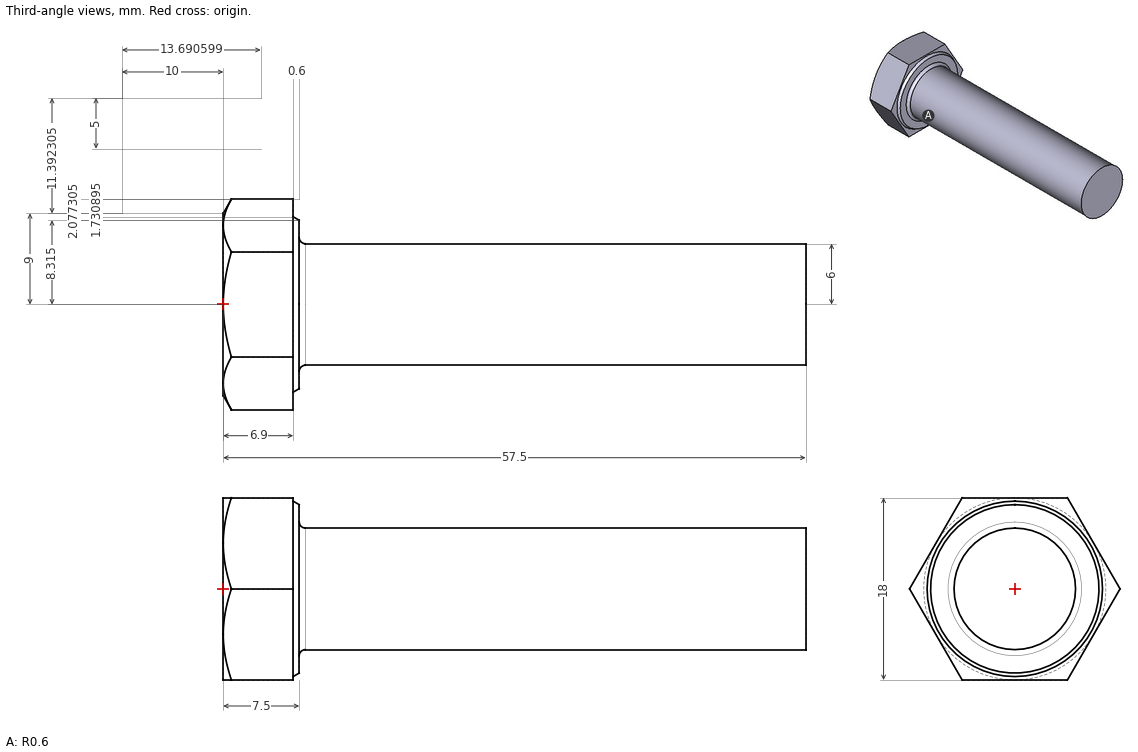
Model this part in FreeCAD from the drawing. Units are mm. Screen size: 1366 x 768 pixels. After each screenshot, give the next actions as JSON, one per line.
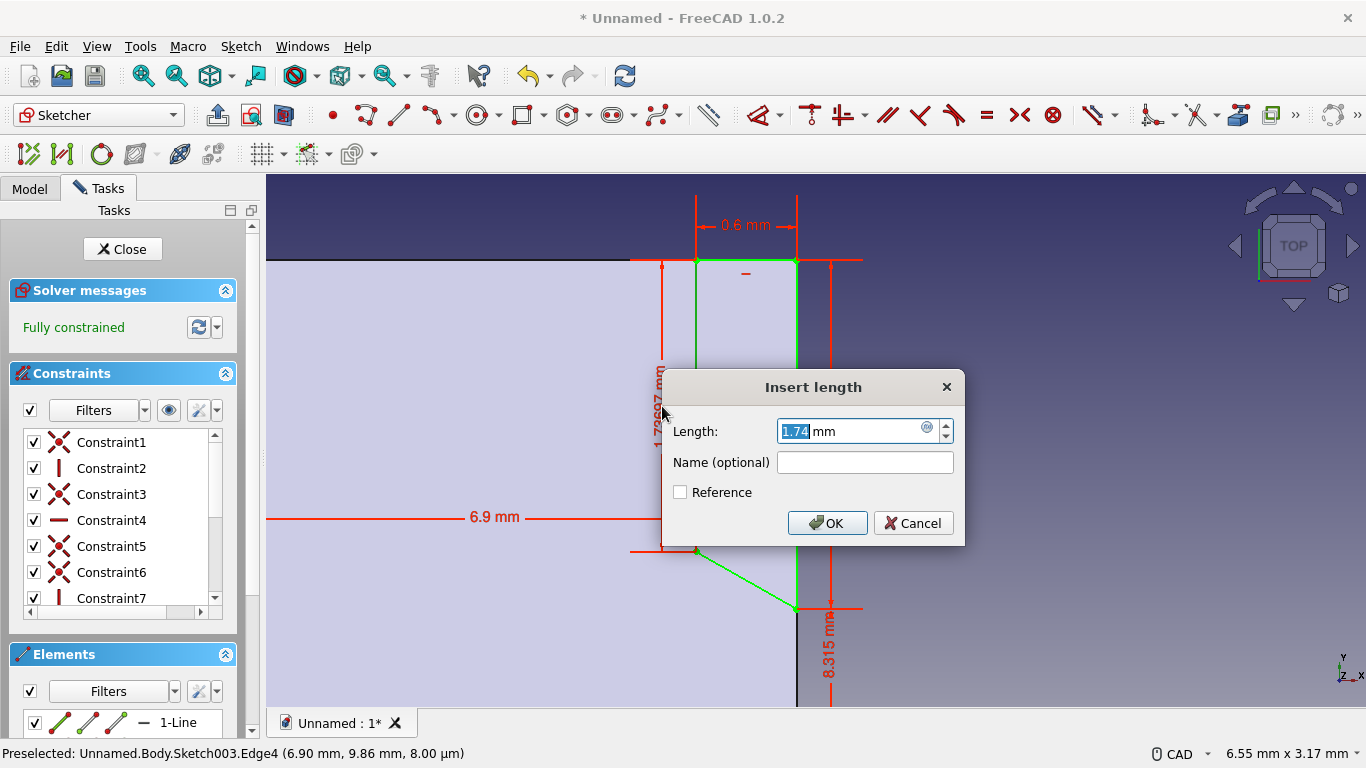
{"action": "type", "text": "1.730895"}
{"action": "key", "text": "Return"}
{"action": "key", "text": "Escape"}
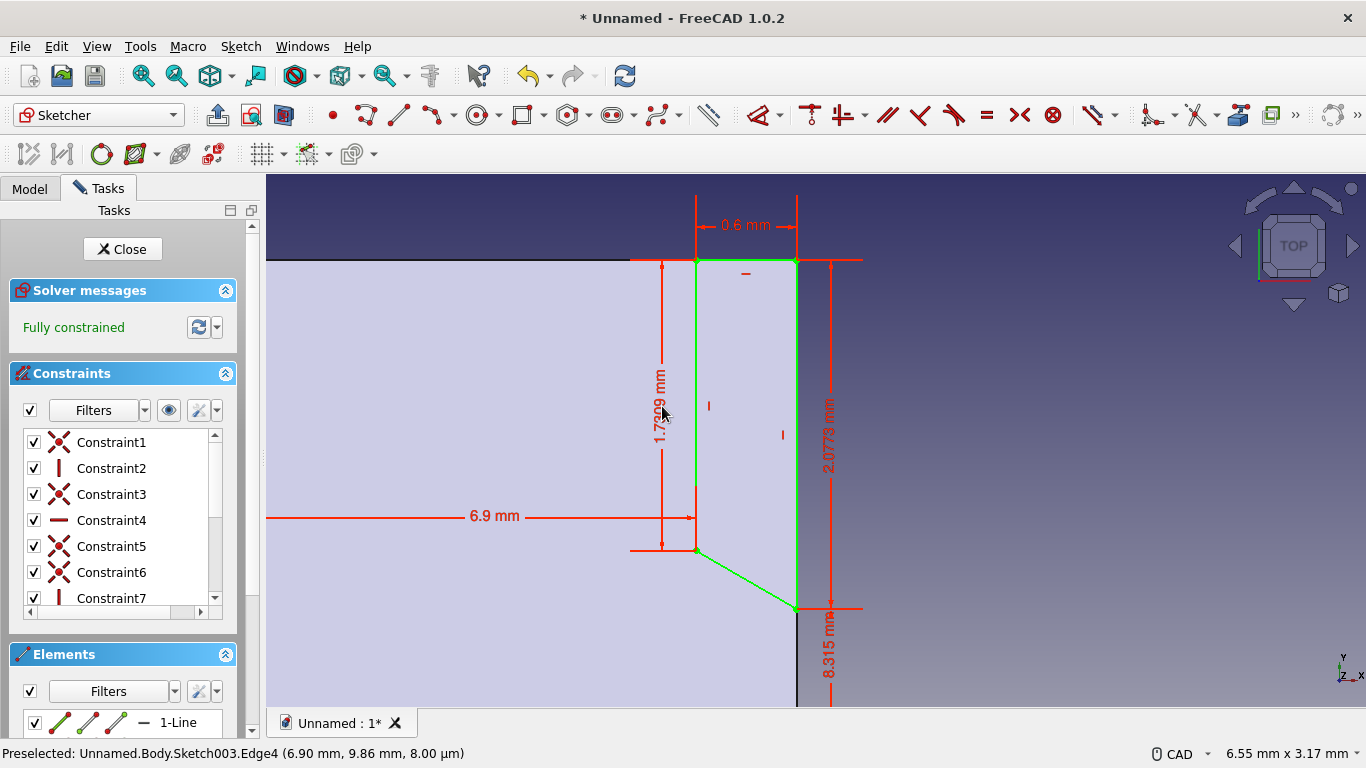
{"action": "left_click", "coordinate": [123, 249]}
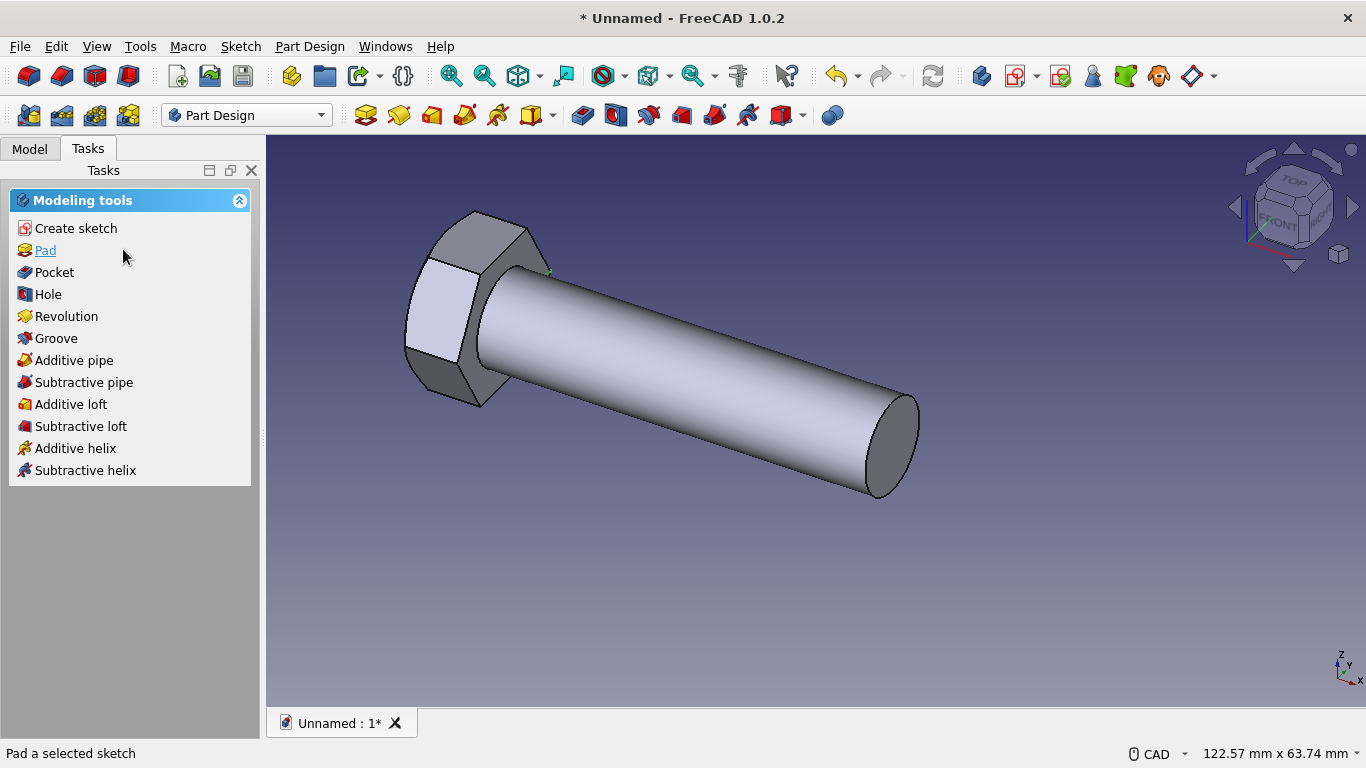
{"action": "left_click", "coordinate": [649, 116]}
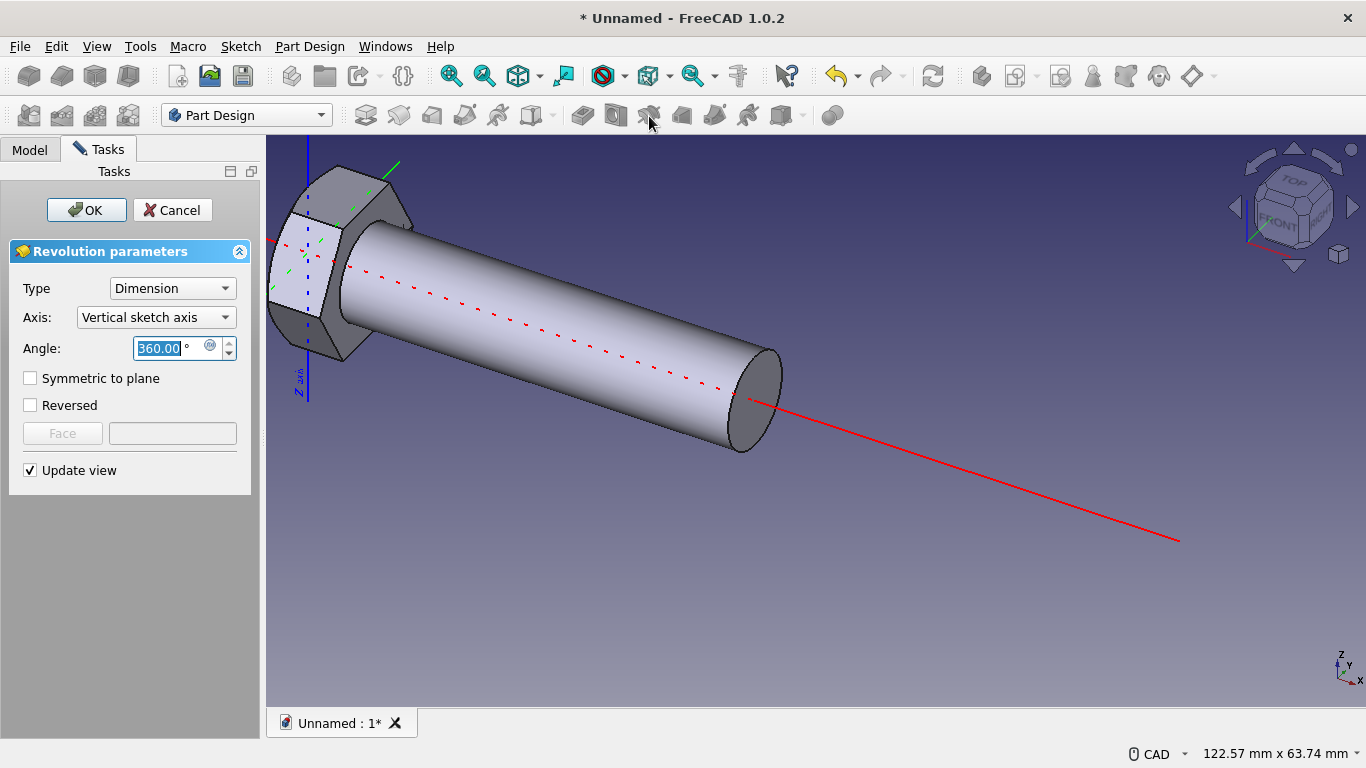
{"action": "left_click", "coordinate": [157, 318]}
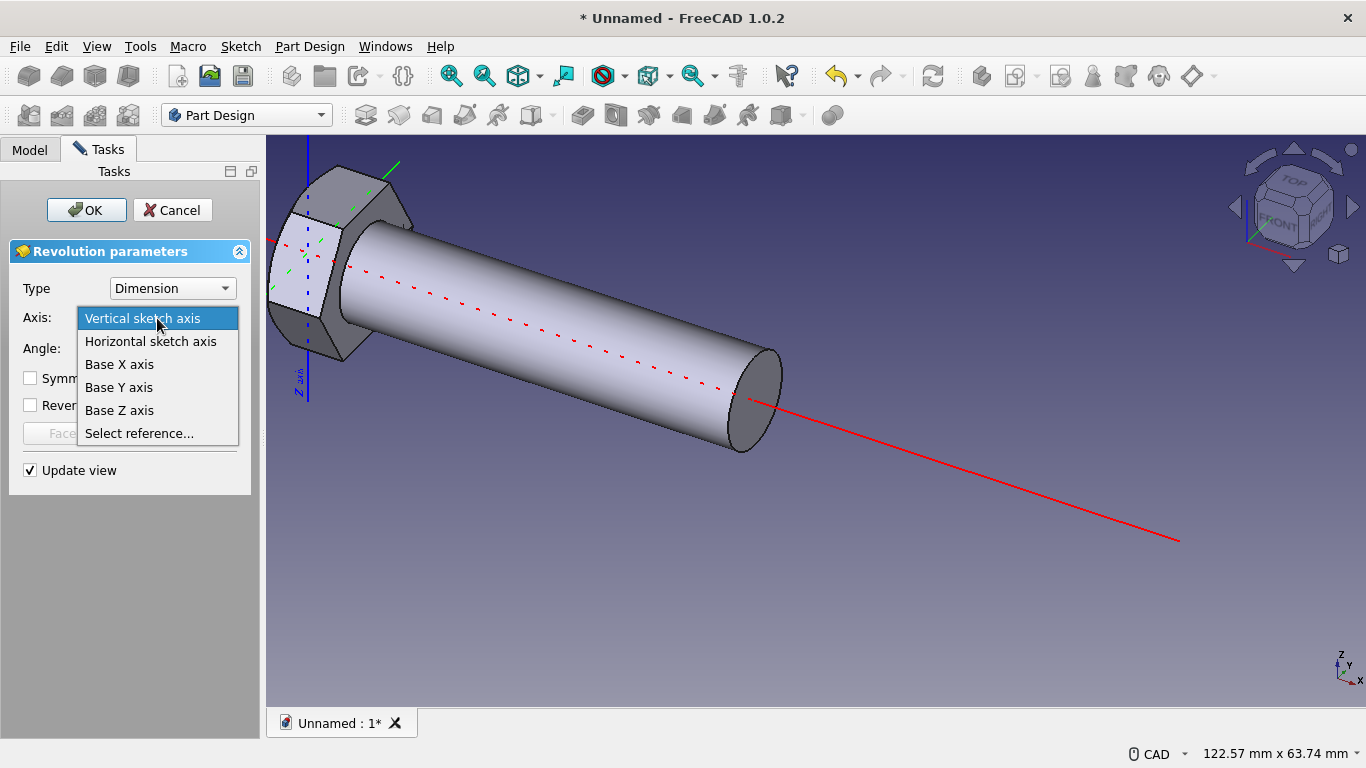
{"action": "left_click", "coordinate": [156, 342]}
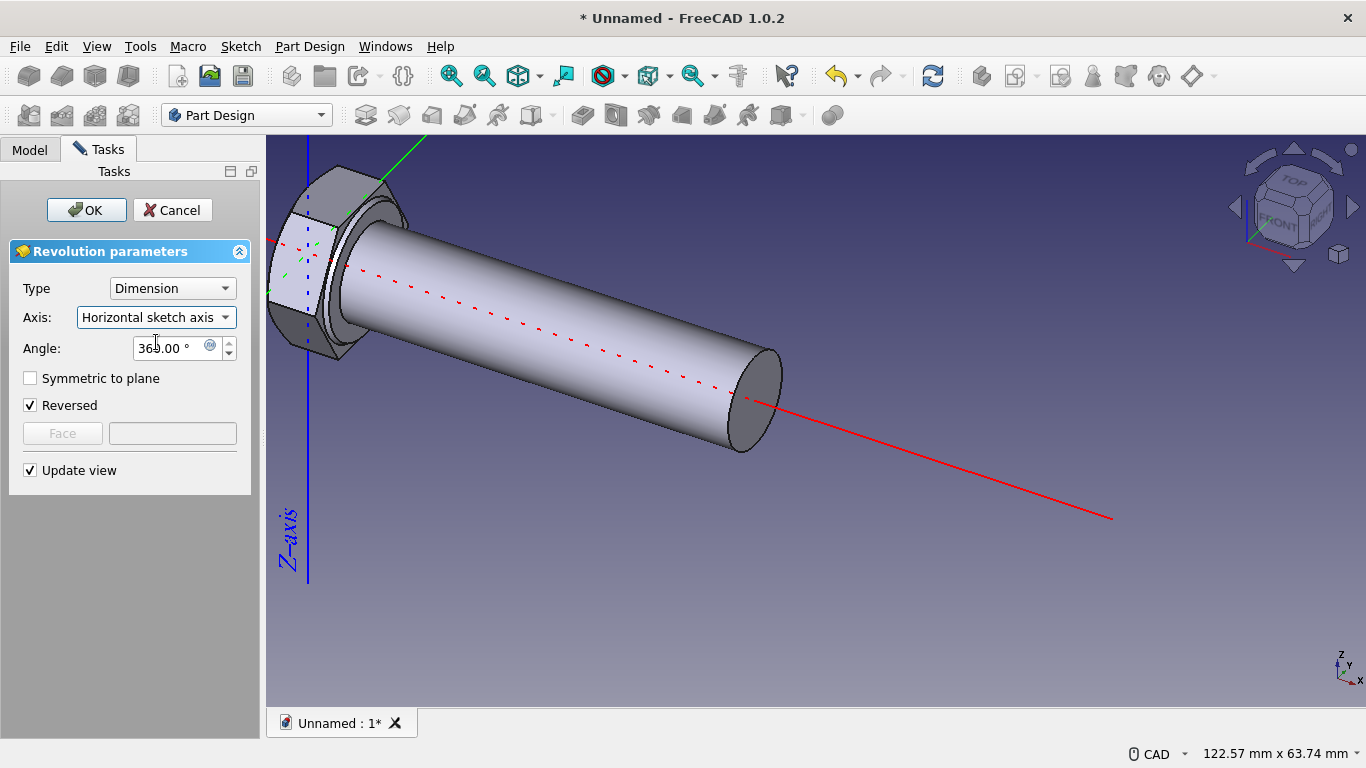
{"action": "left_click", "coordinate": [87, 210]}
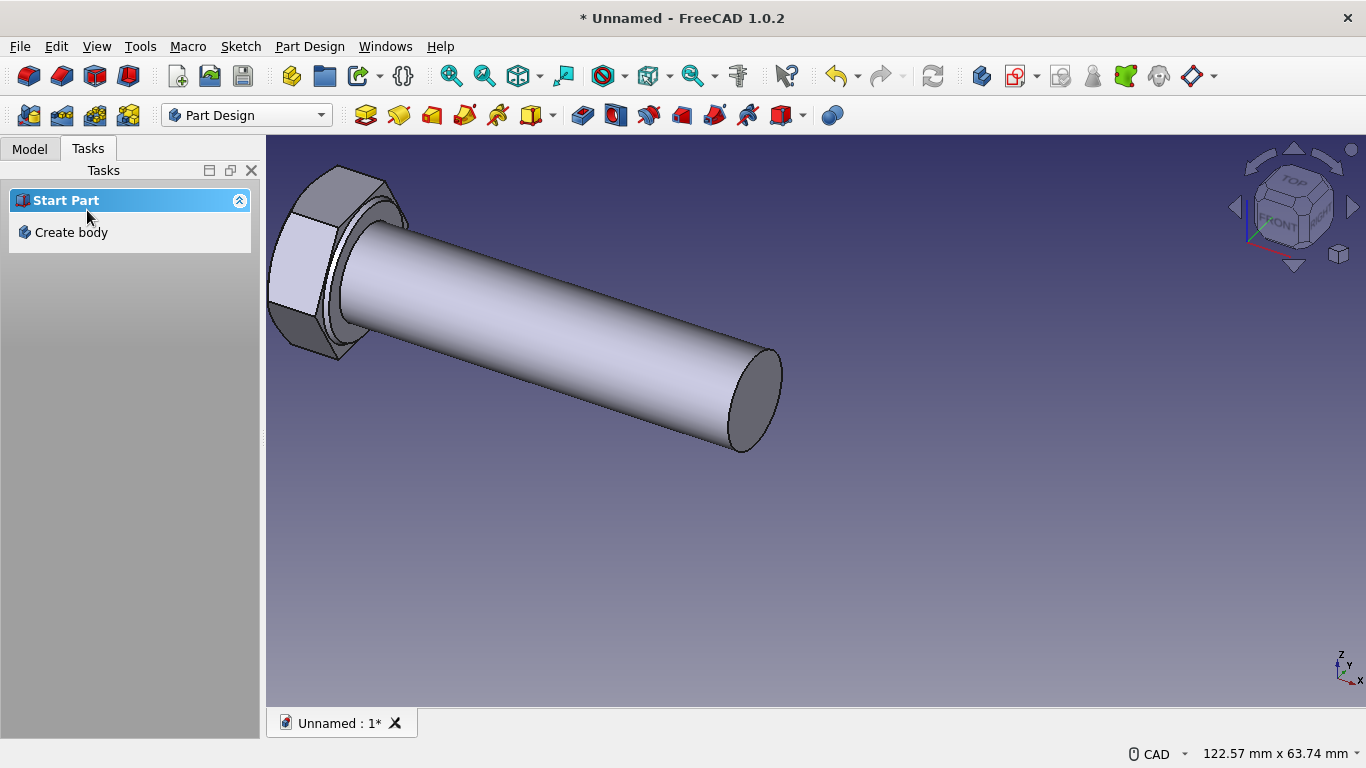
{"action": "left_click", "coordinate": [452, 76]}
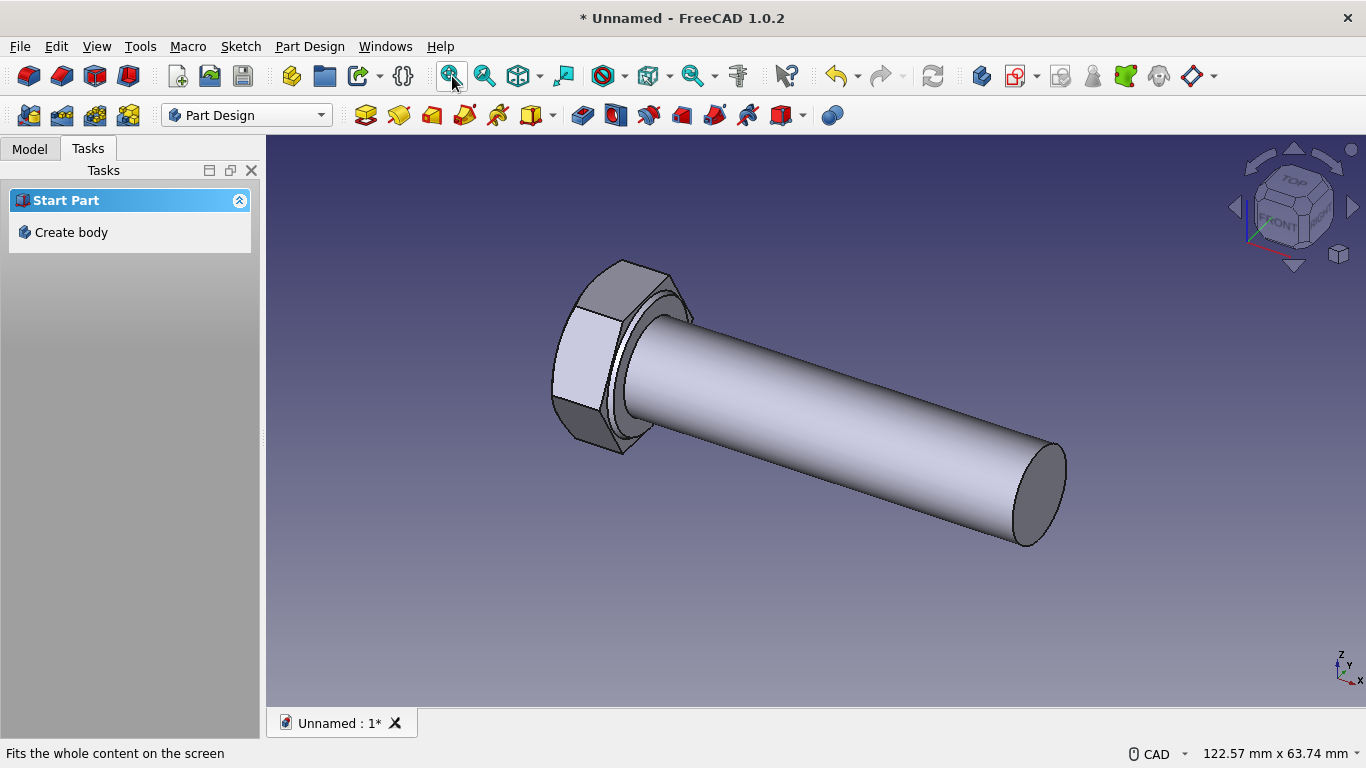
{"action": "key", "text": "0"}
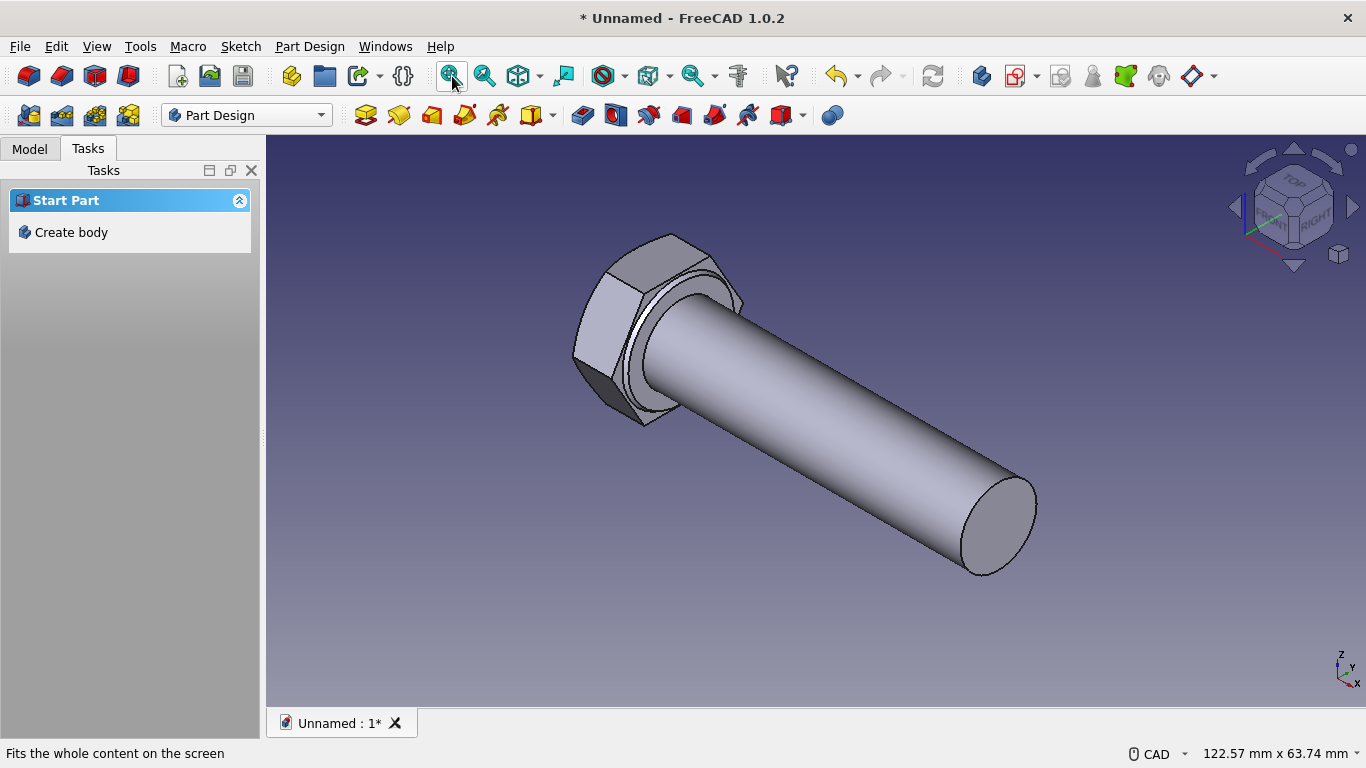
{"action": "key", "text": "2"}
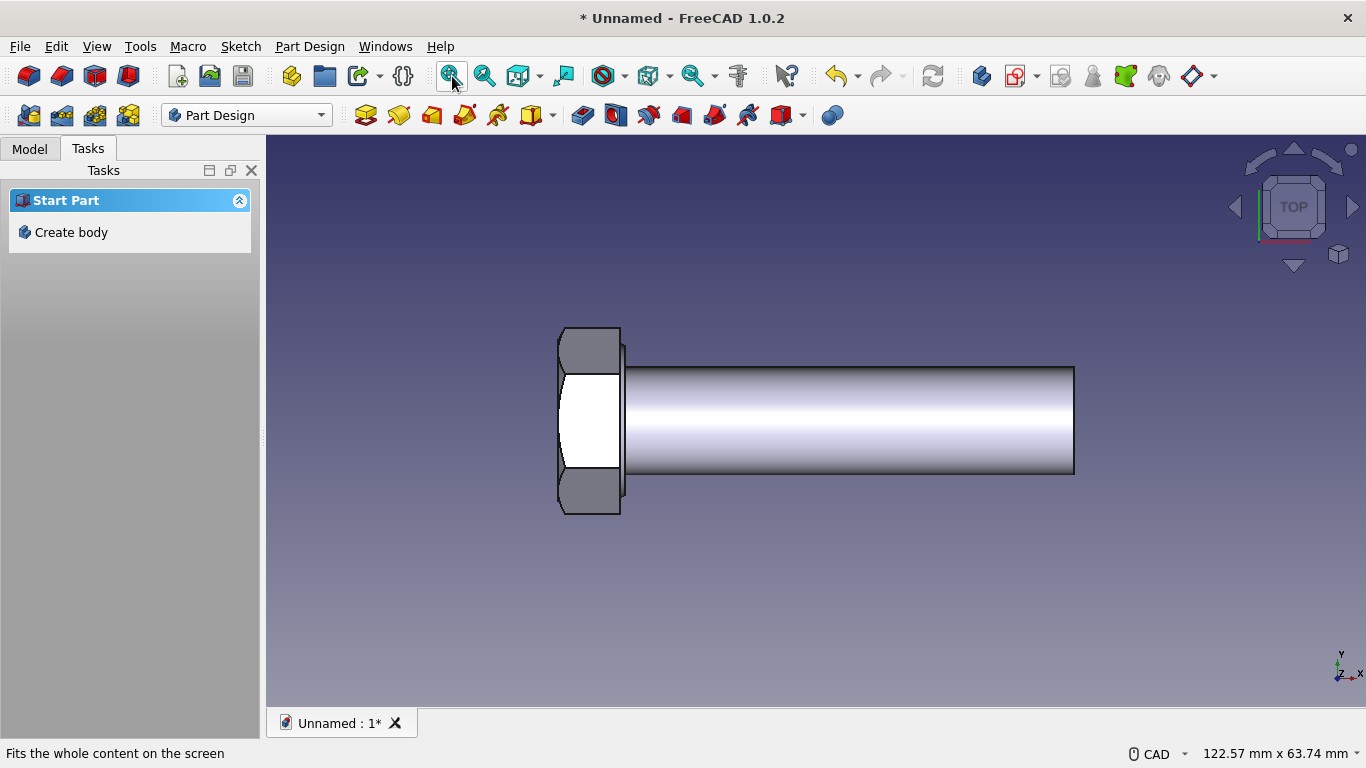
{"action": "key", "text": "1"}